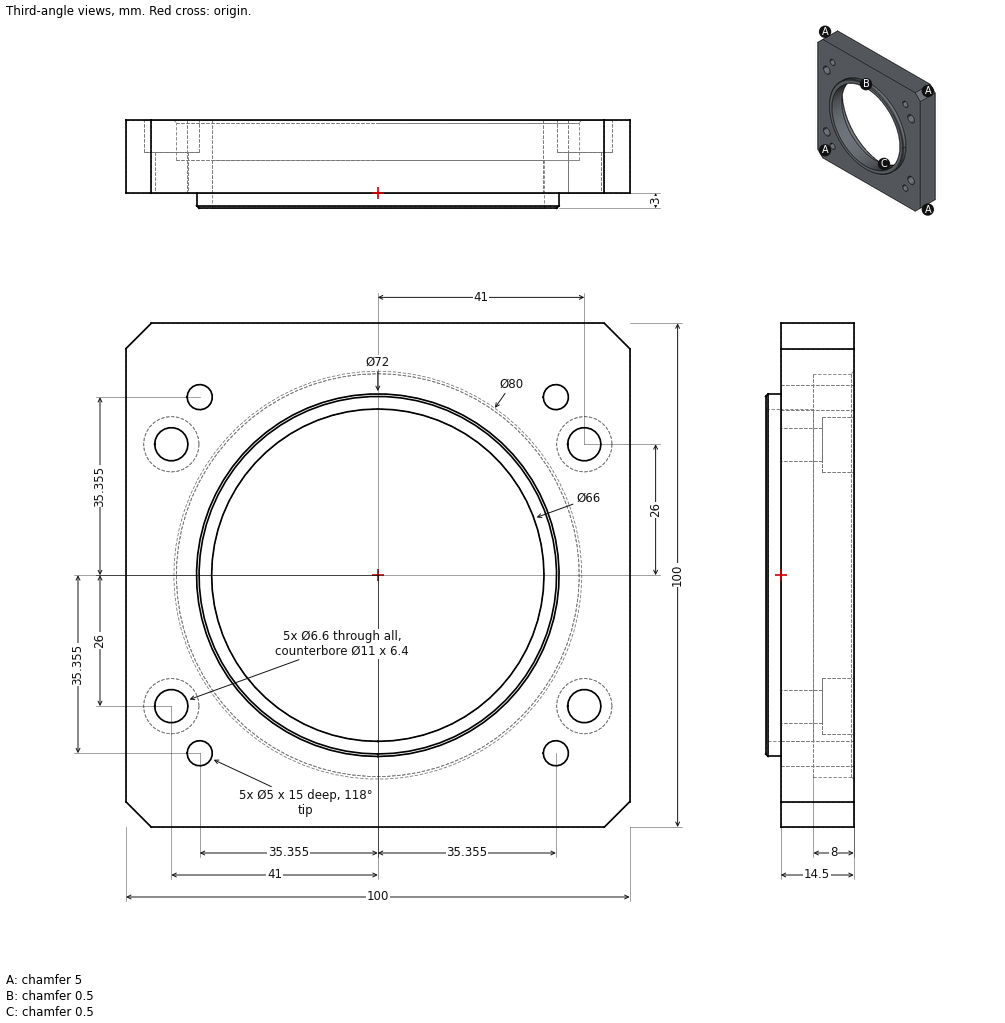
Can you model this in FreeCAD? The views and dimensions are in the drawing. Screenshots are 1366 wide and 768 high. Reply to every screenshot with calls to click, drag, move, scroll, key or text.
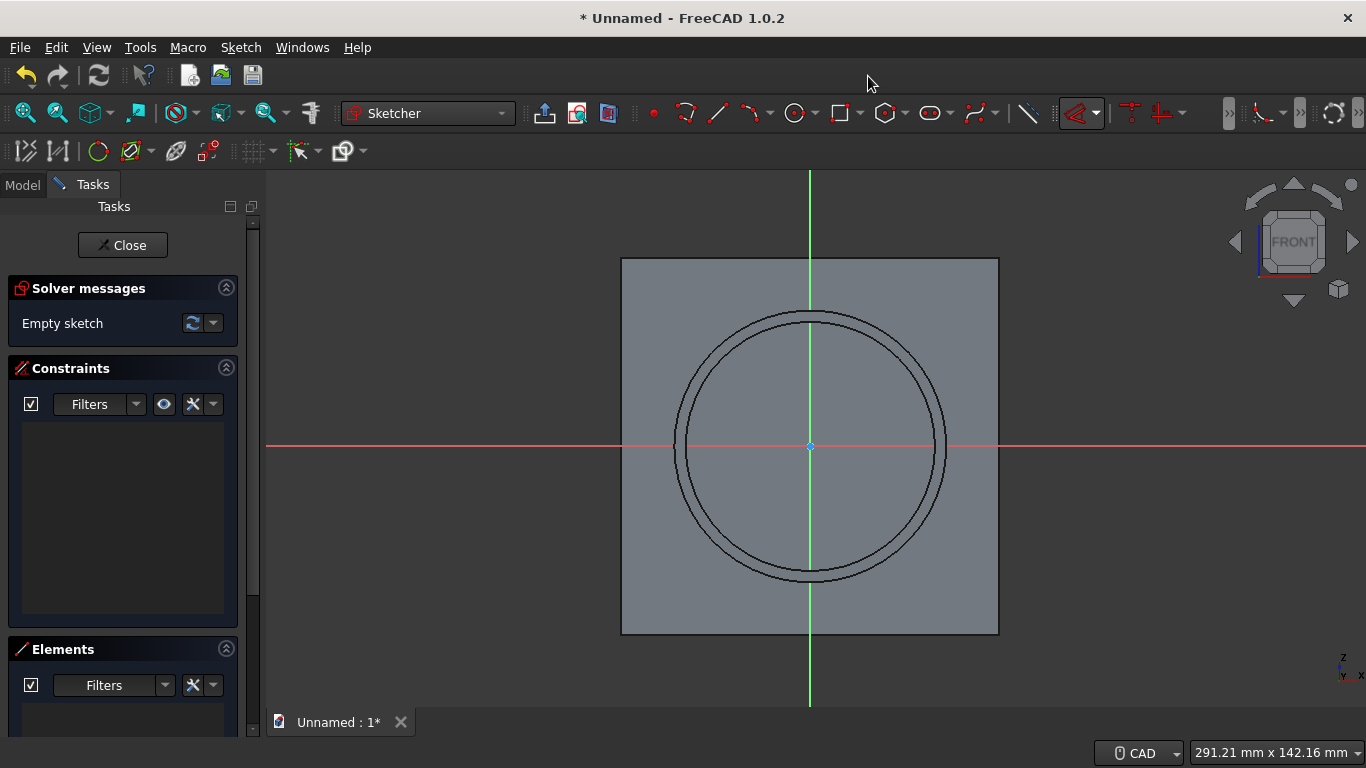
scroll(938, 463, up, 2)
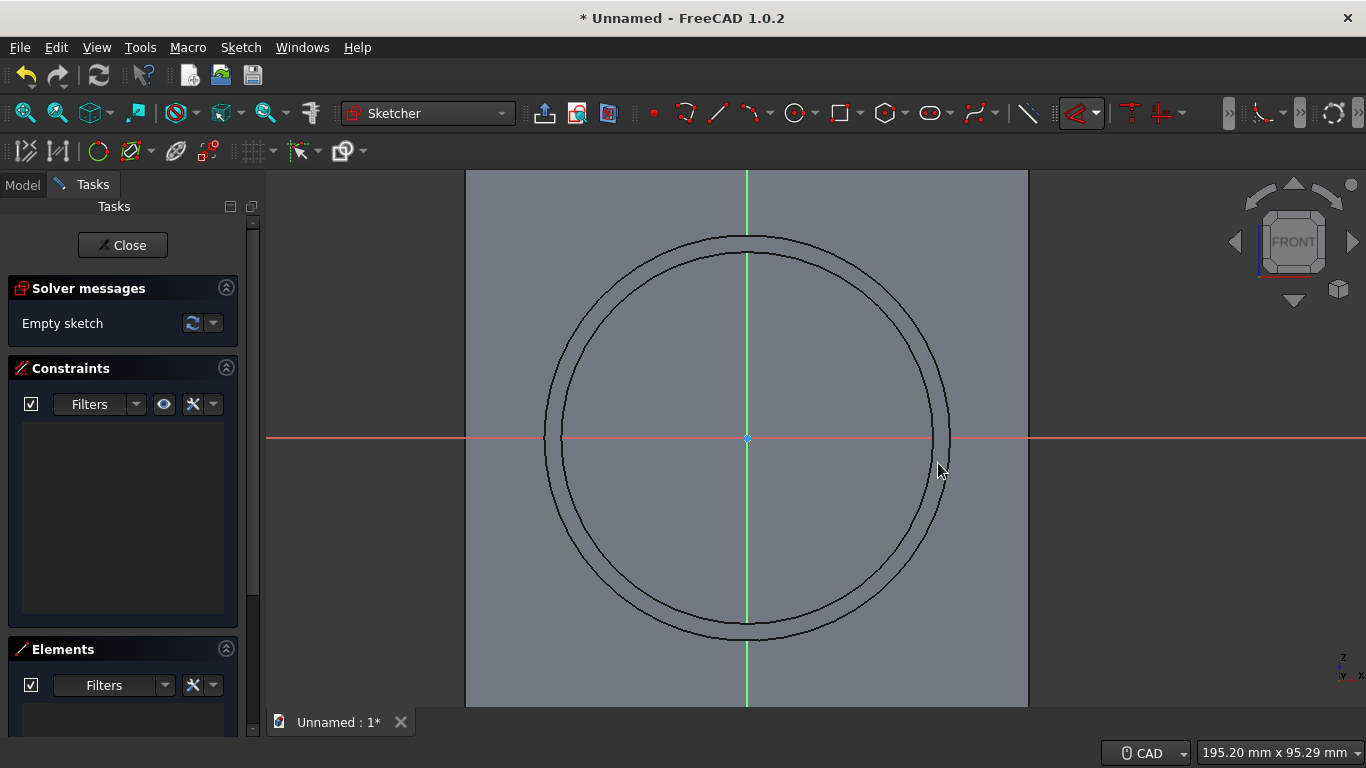
key(g)
key(c)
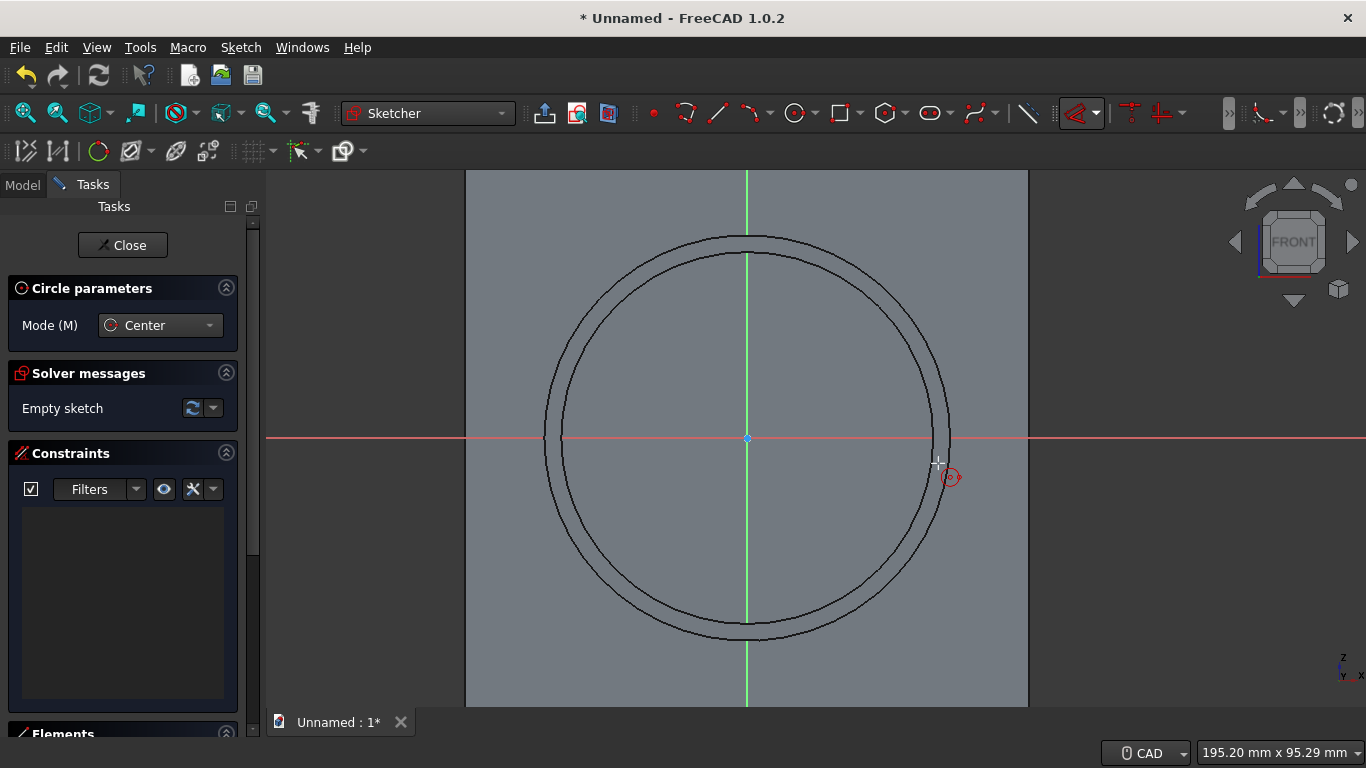
click(747, 438)
click(879, 307)
key(Escape)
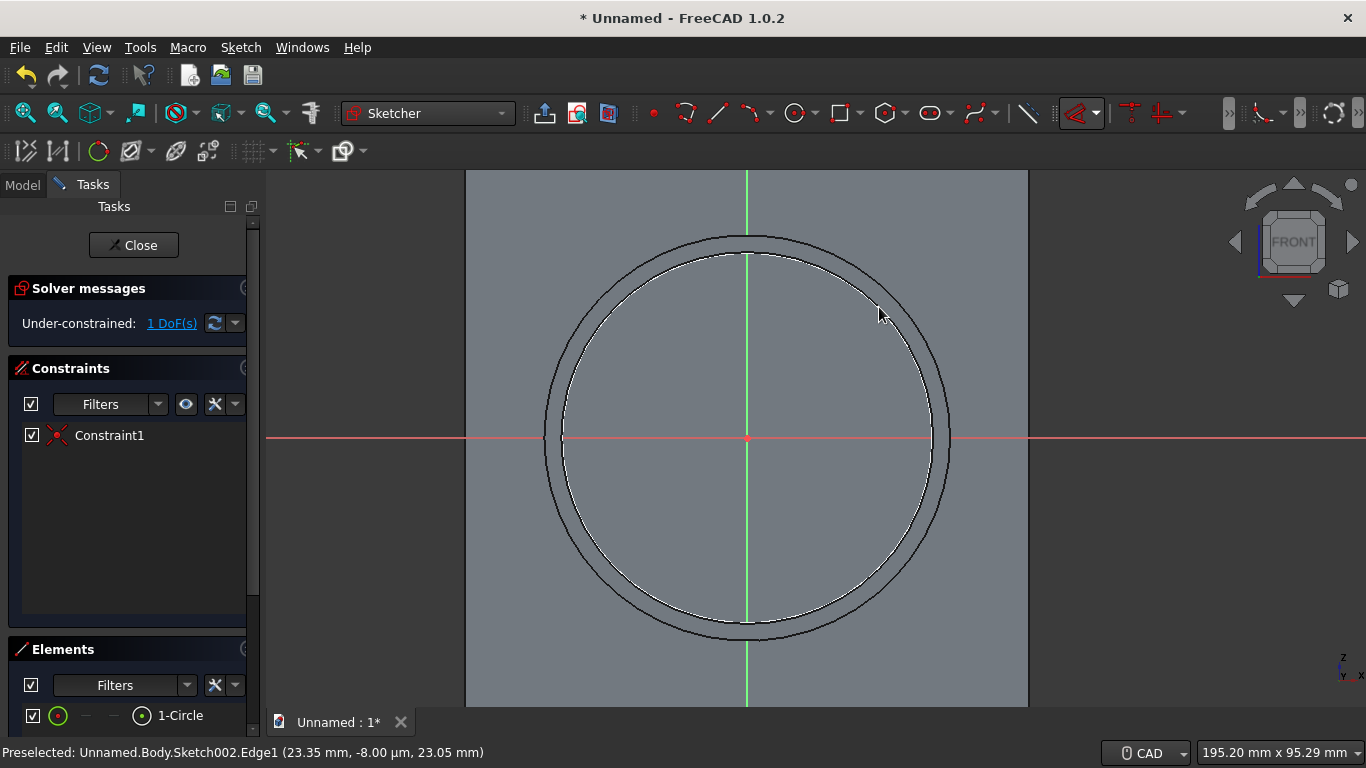
key(d)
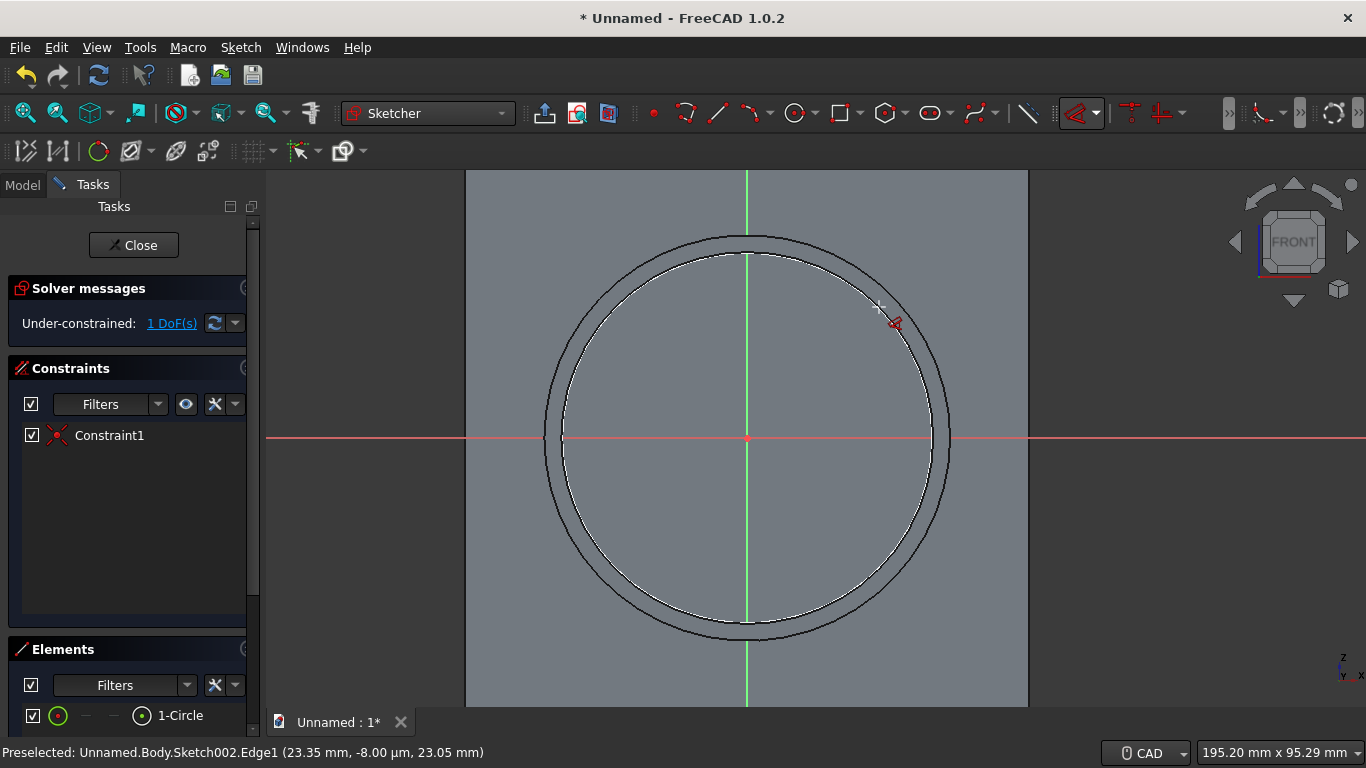
click(878, 307)
click(901, 284)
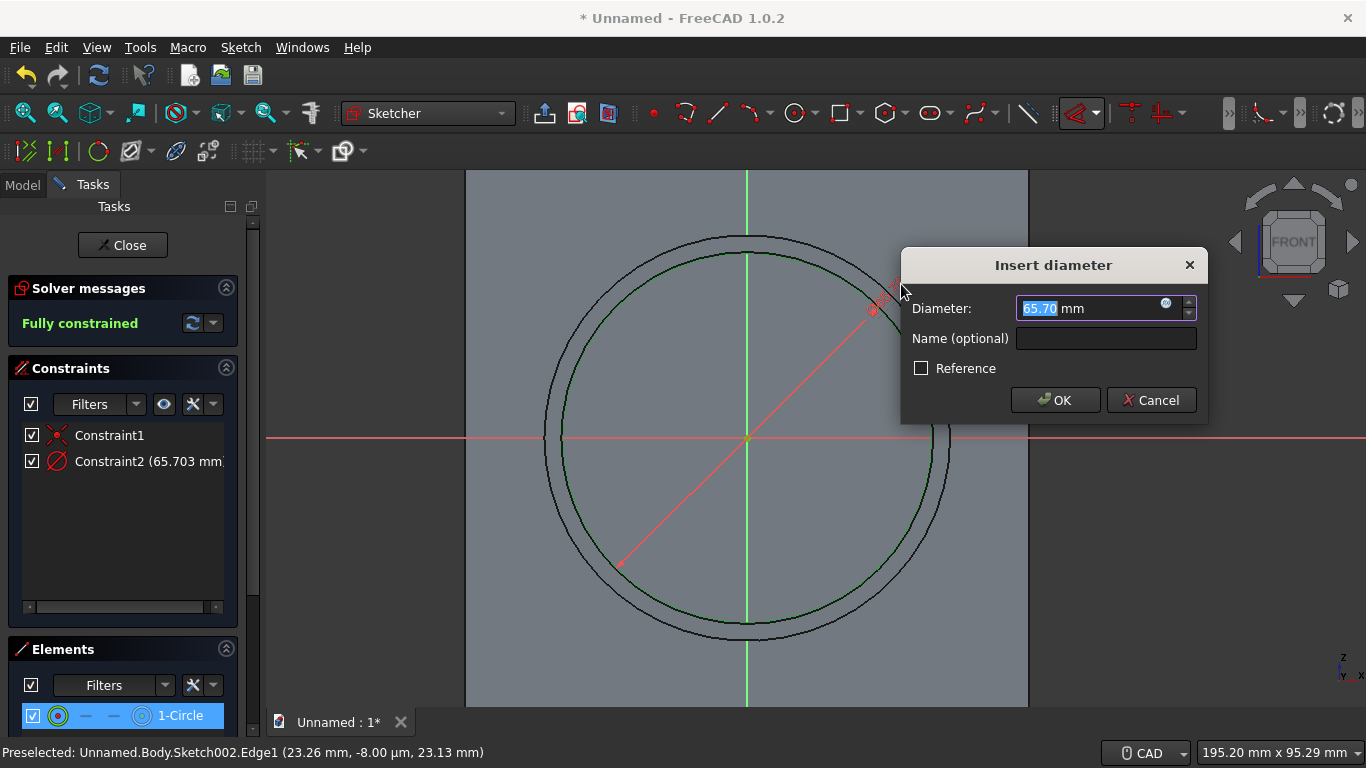
text(66)
key(Return)
key(Escape)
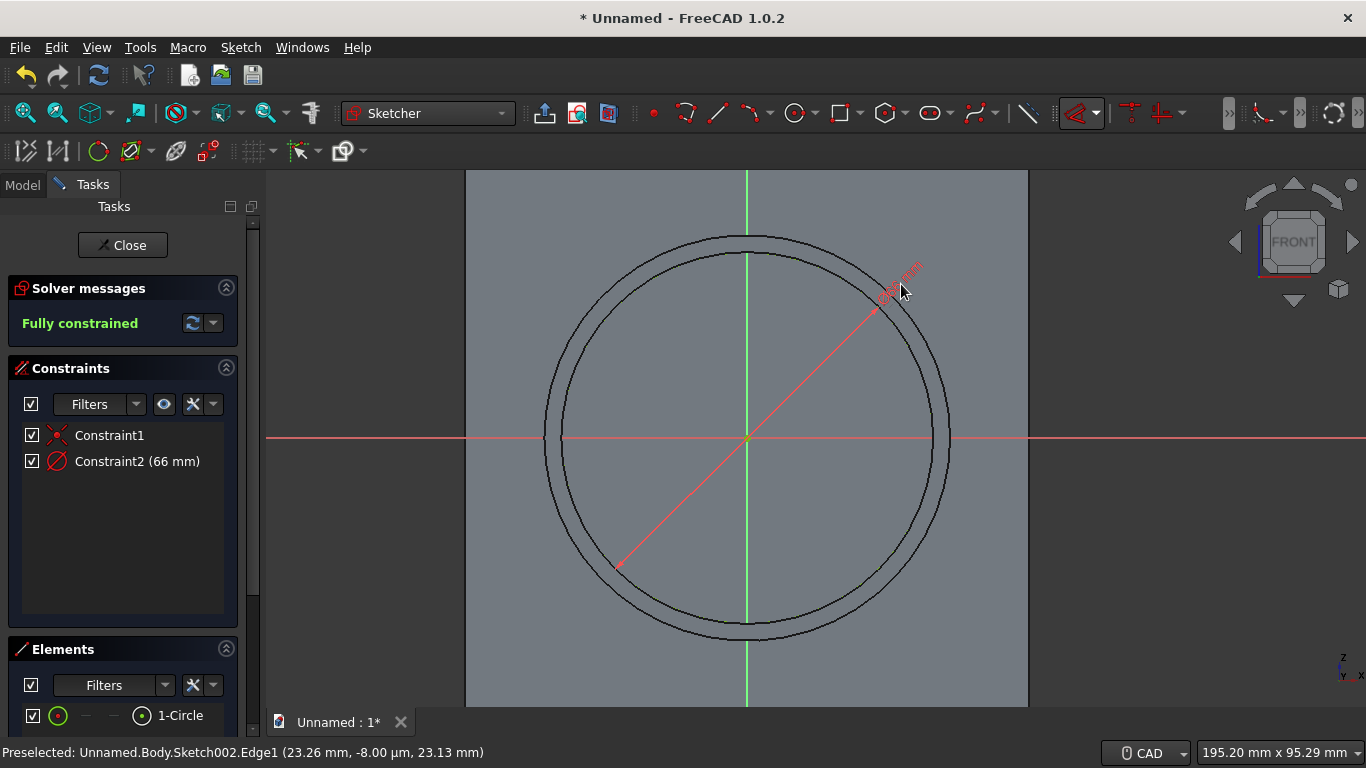
click(123, 245)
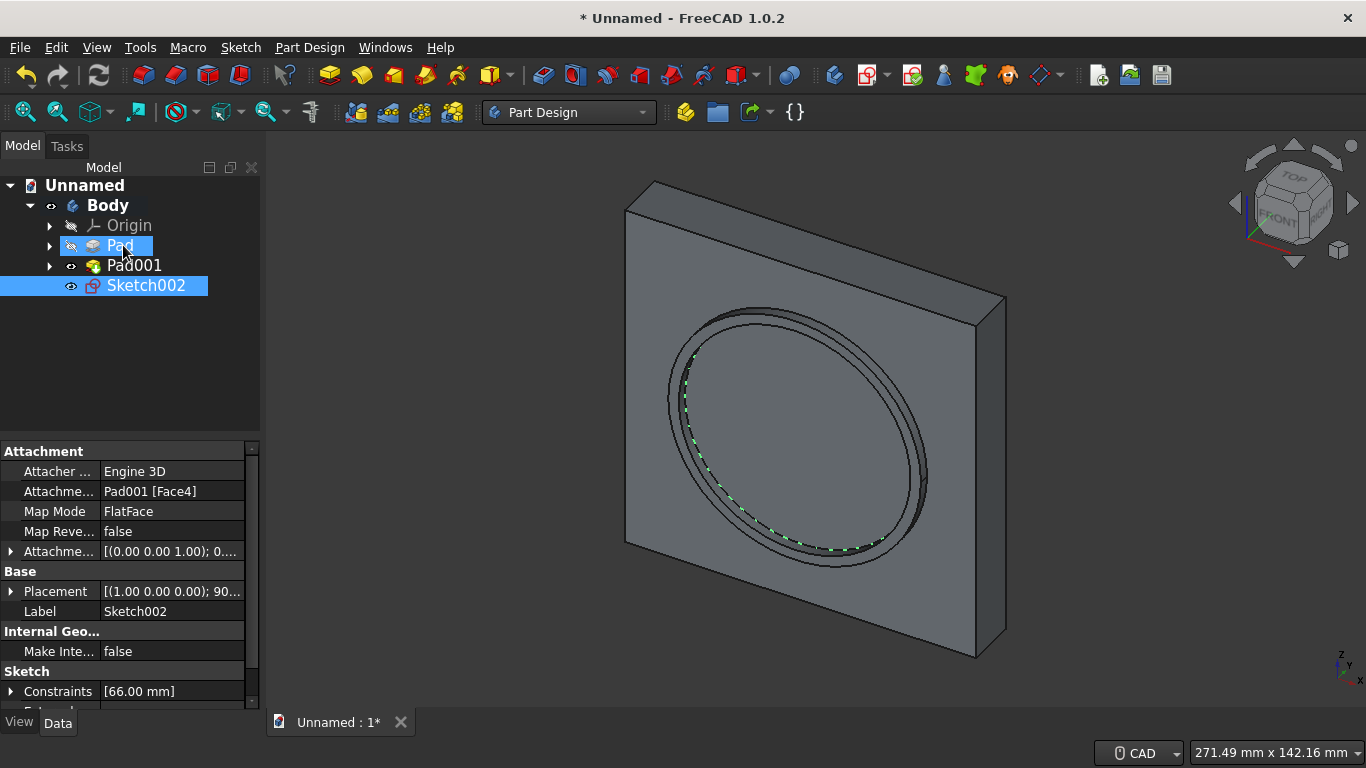
click(544, 76)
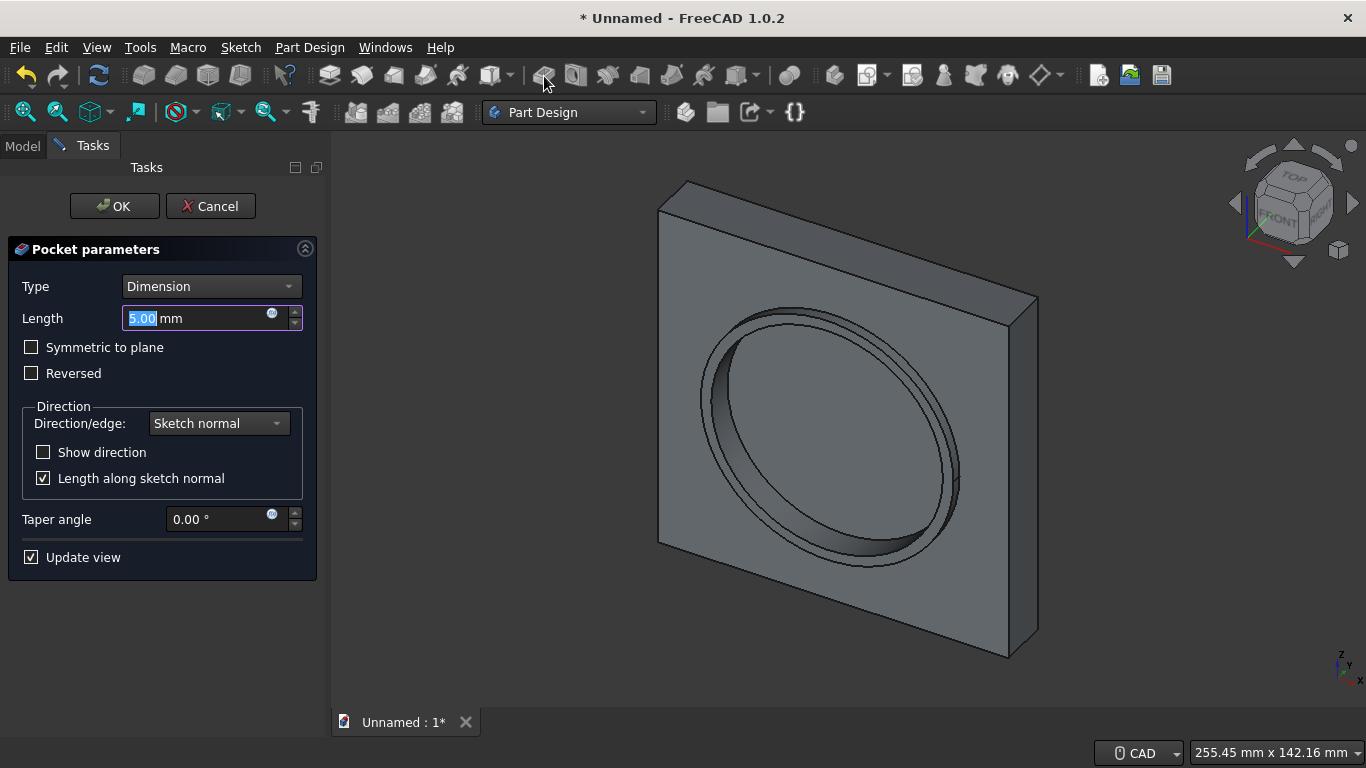
click(212, 286)